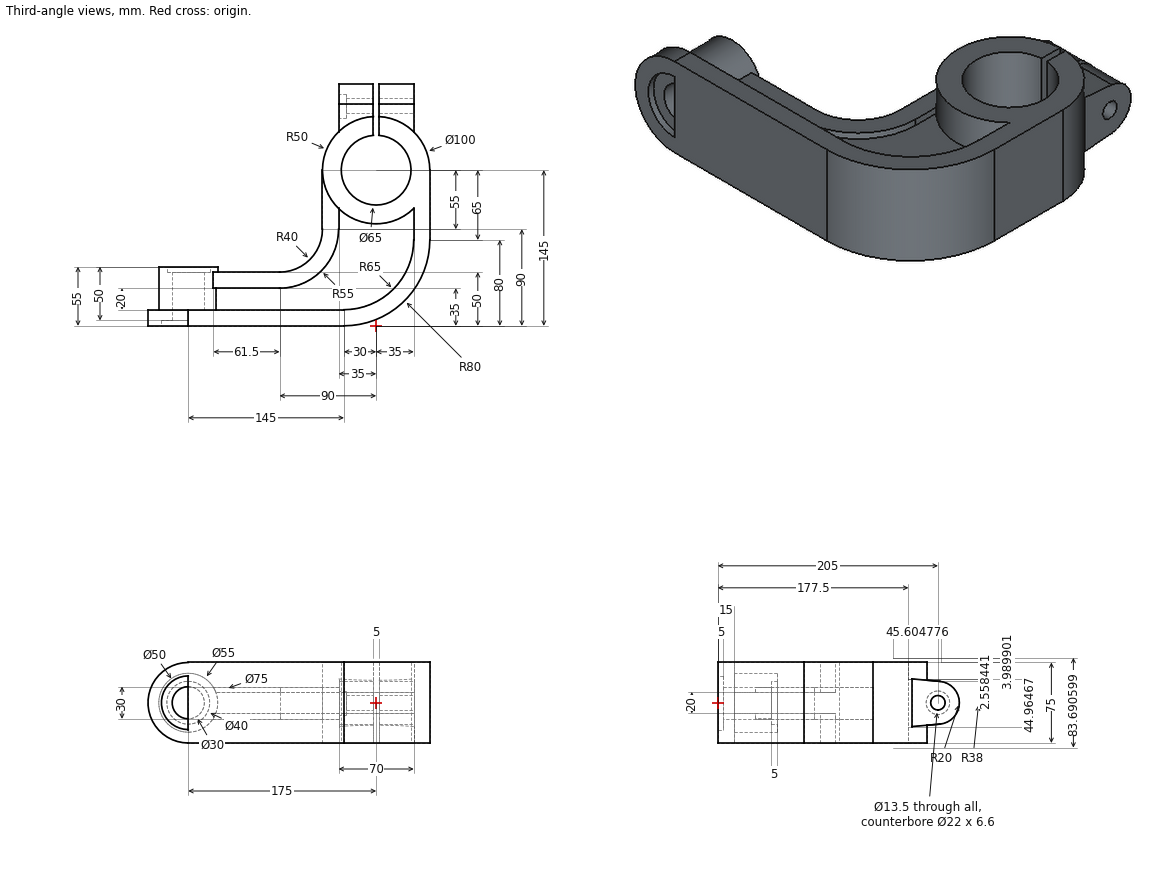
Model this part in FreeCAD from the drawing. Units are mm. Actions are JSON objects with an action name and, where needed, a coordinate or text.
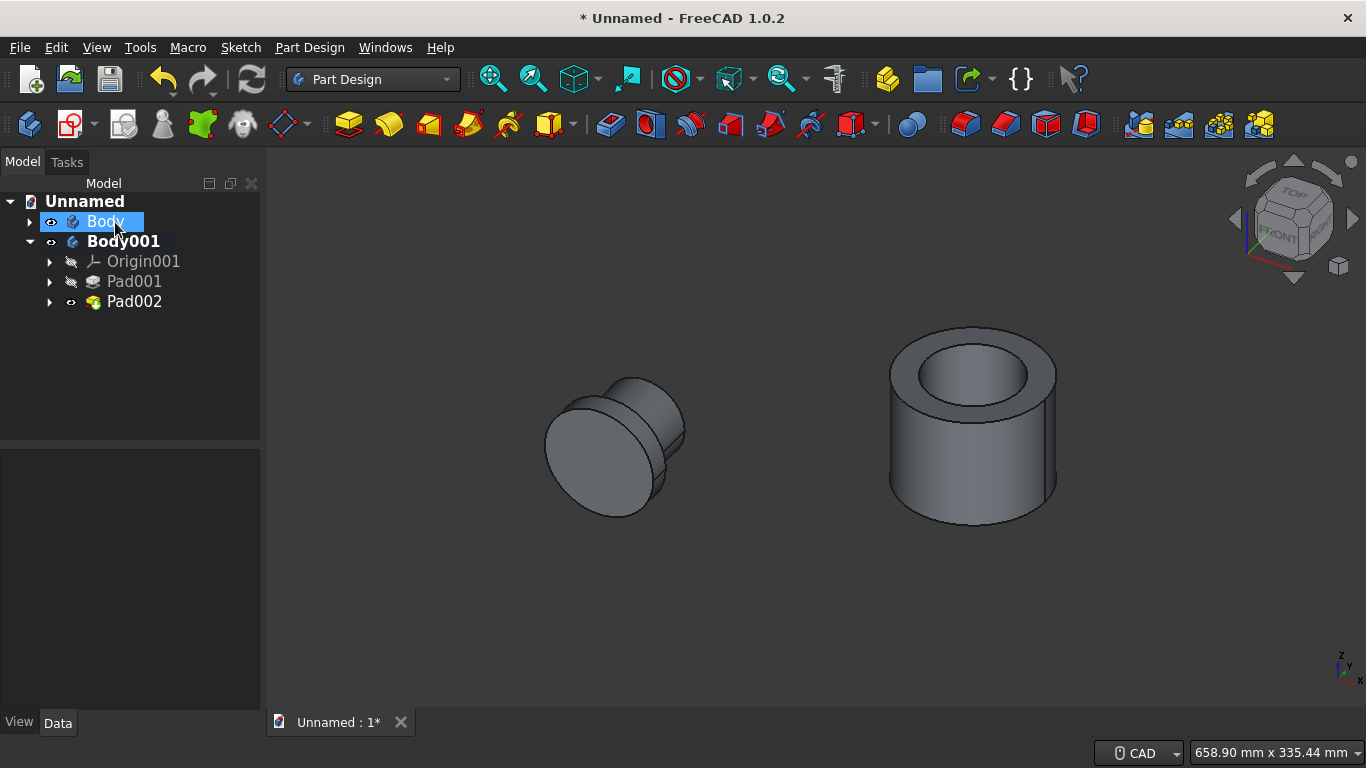
{"action": "left_click", "coordinate": [70, 124]}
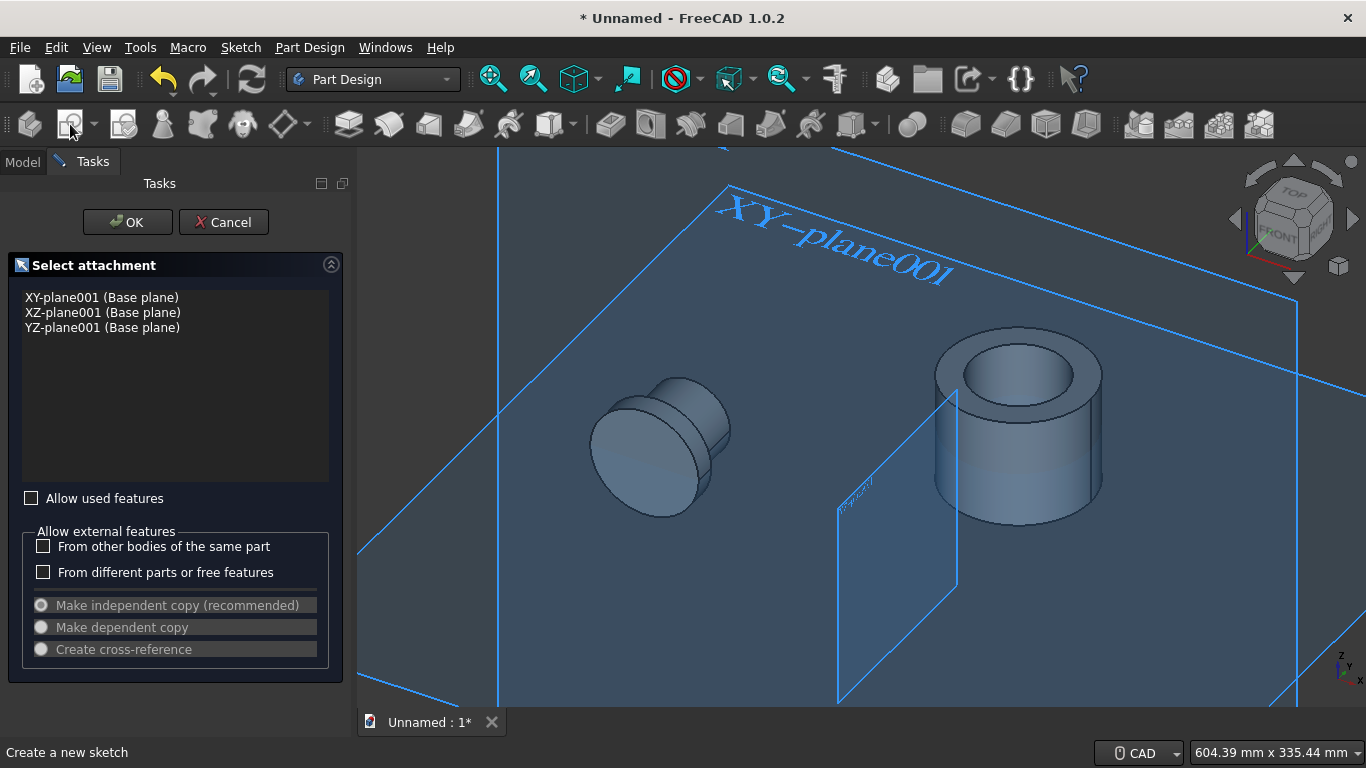
{"action": "left_click", "coordinate": [82, 312]}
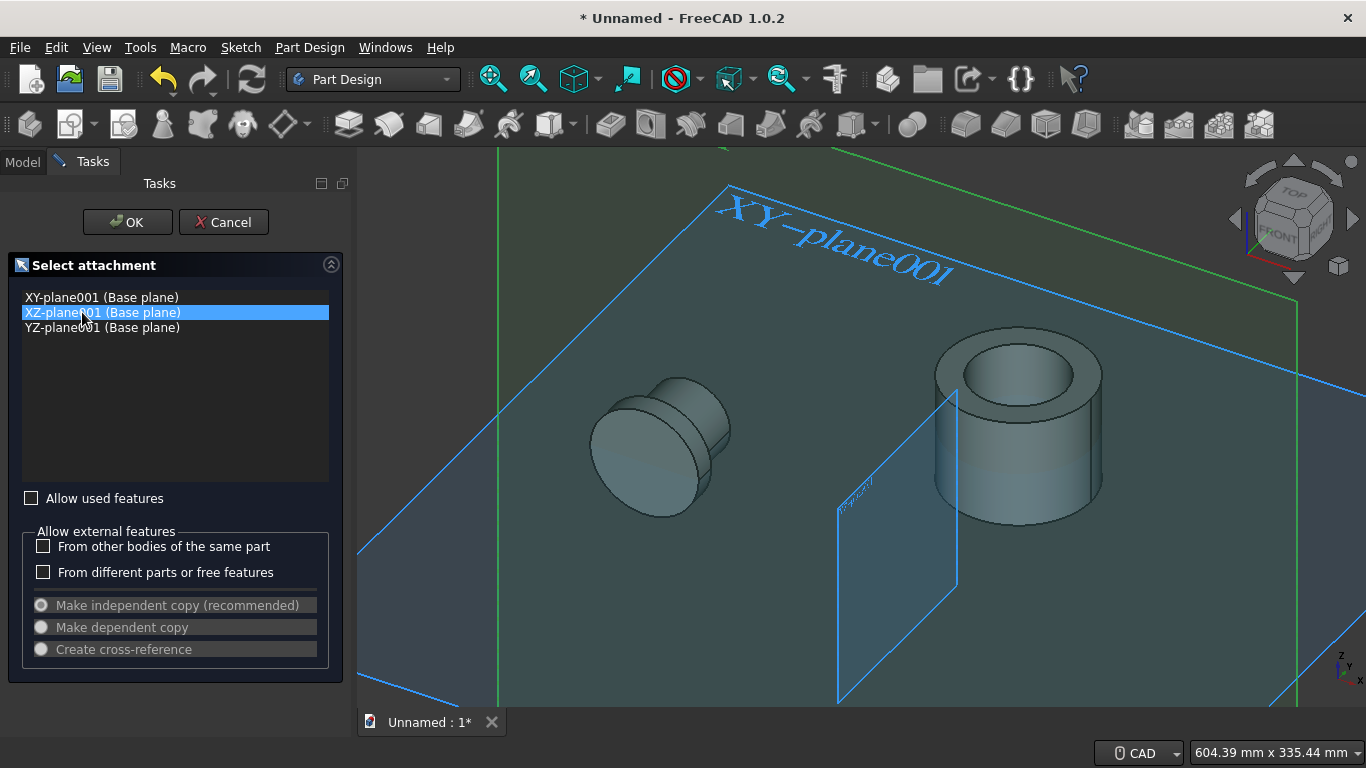
{"action": "left_click", "coordinate": [128, 222]}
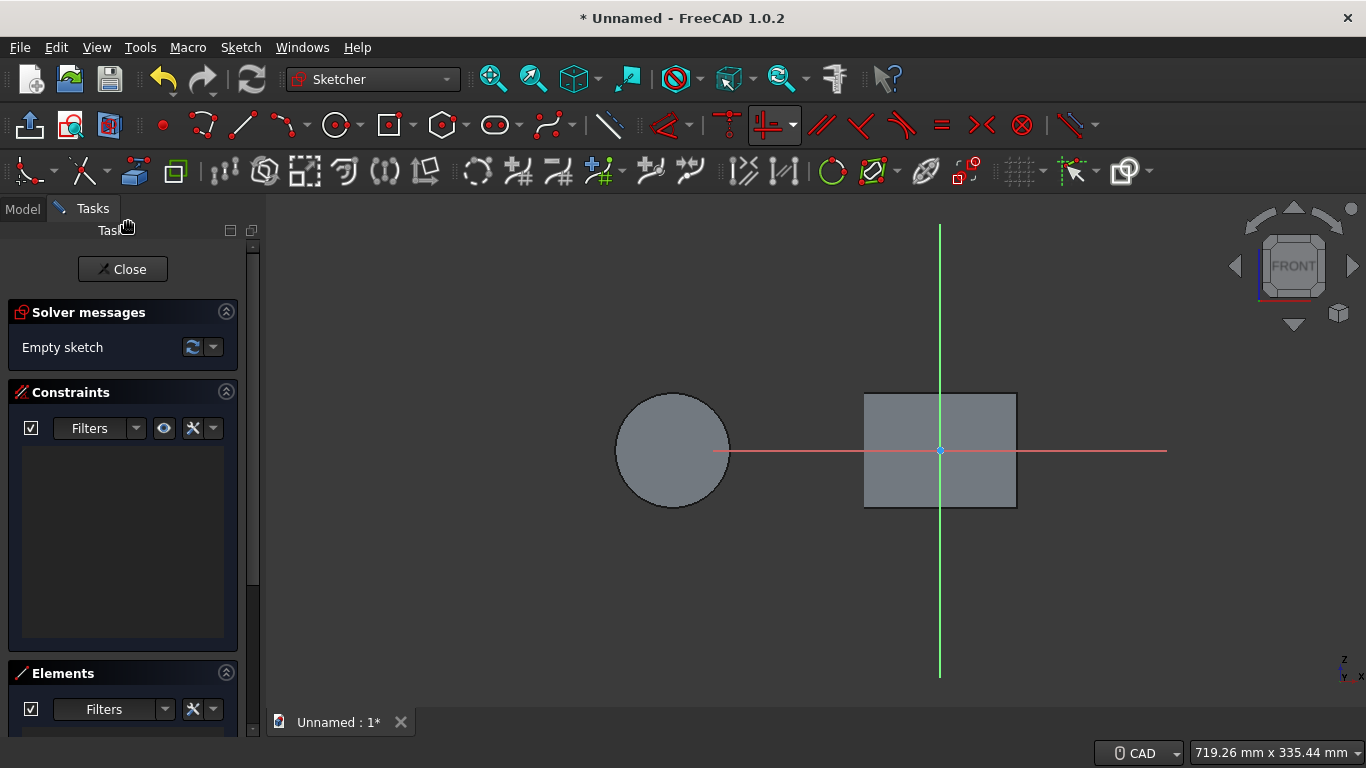
{"action": "scroll", "coordinate": [648, 450], "scroll_direction": "up", "scroll_amount": 7}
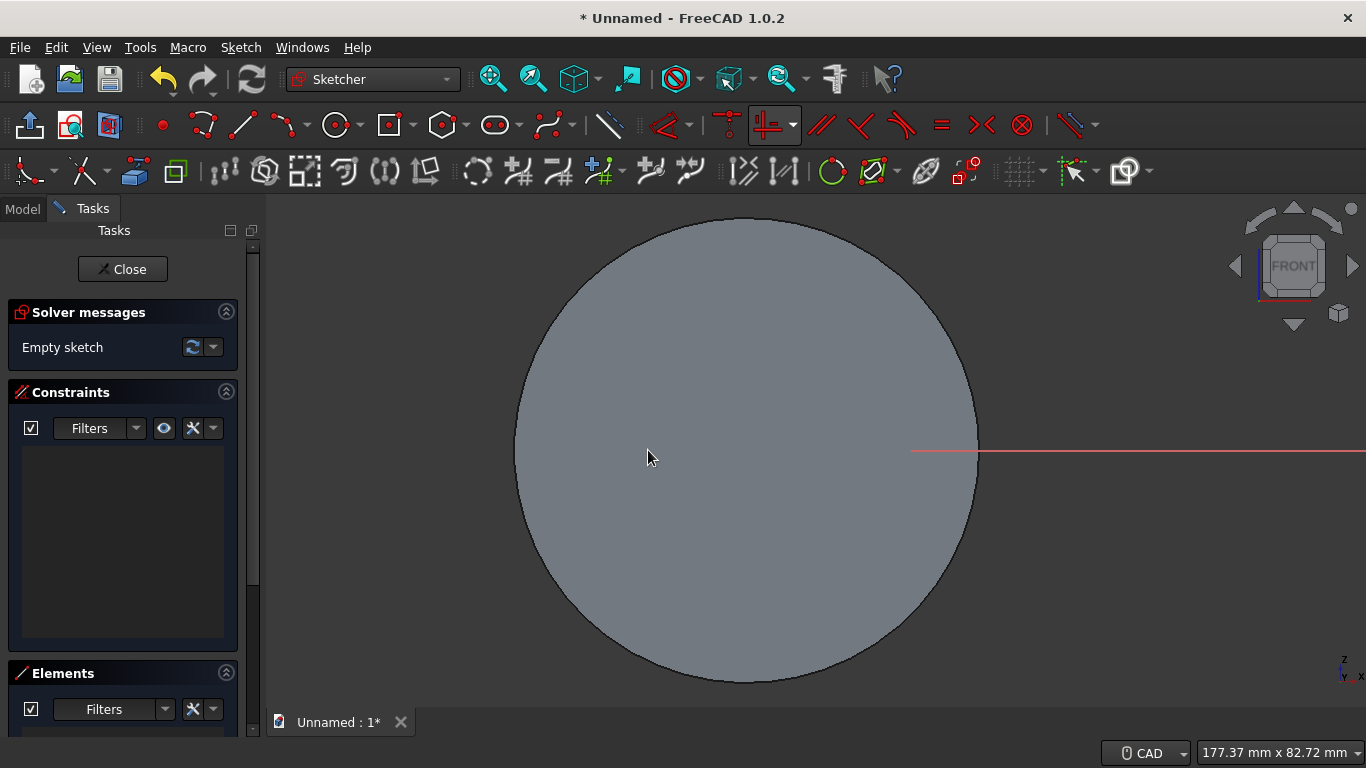
{"action": "key", "text": "g c"}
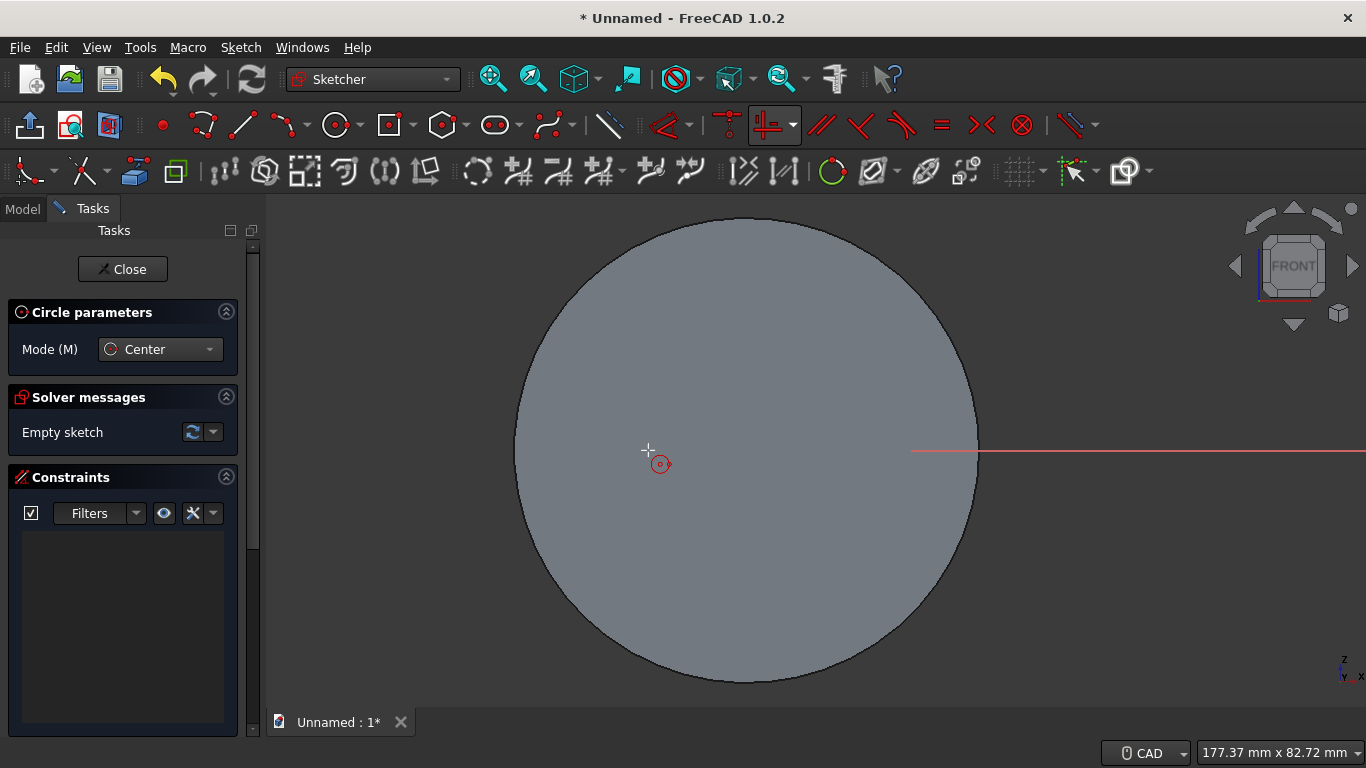
{"action": "left_click", "coordinate": [747, 450]}
{"action": "left_click", "coordinate": [856, 341]}
{"action": "key", "text": "Escape"}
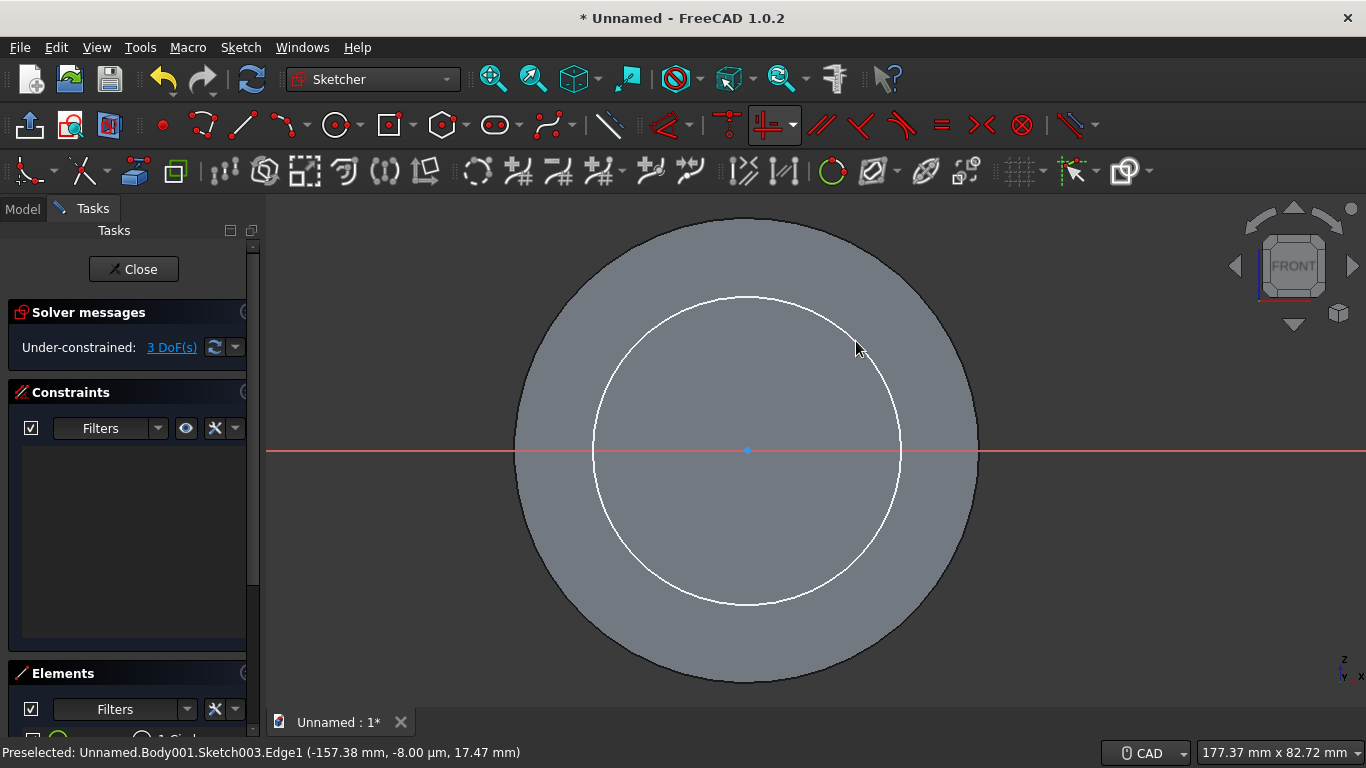
{"action": "left_click", "coordinate": [747, 451]}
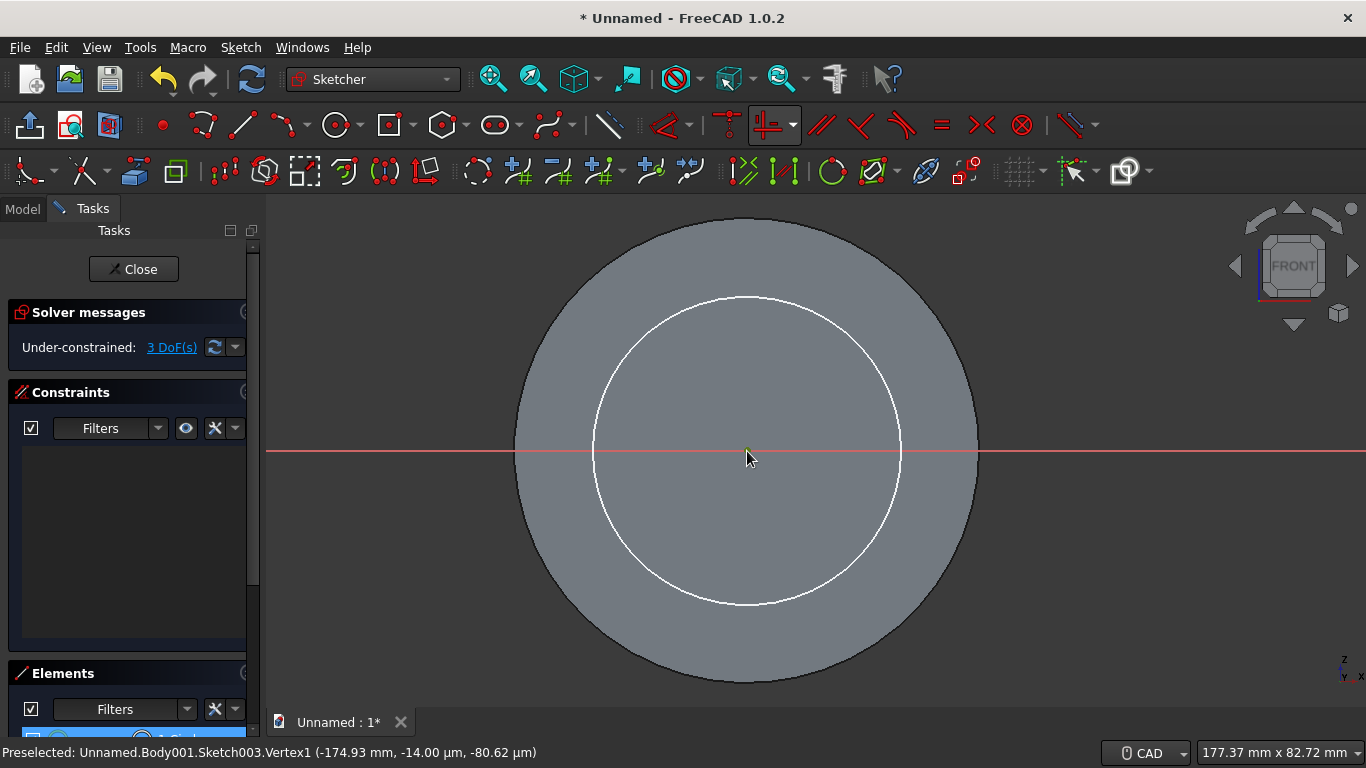
{"action": "left_click", "coordinate": [359, 450]}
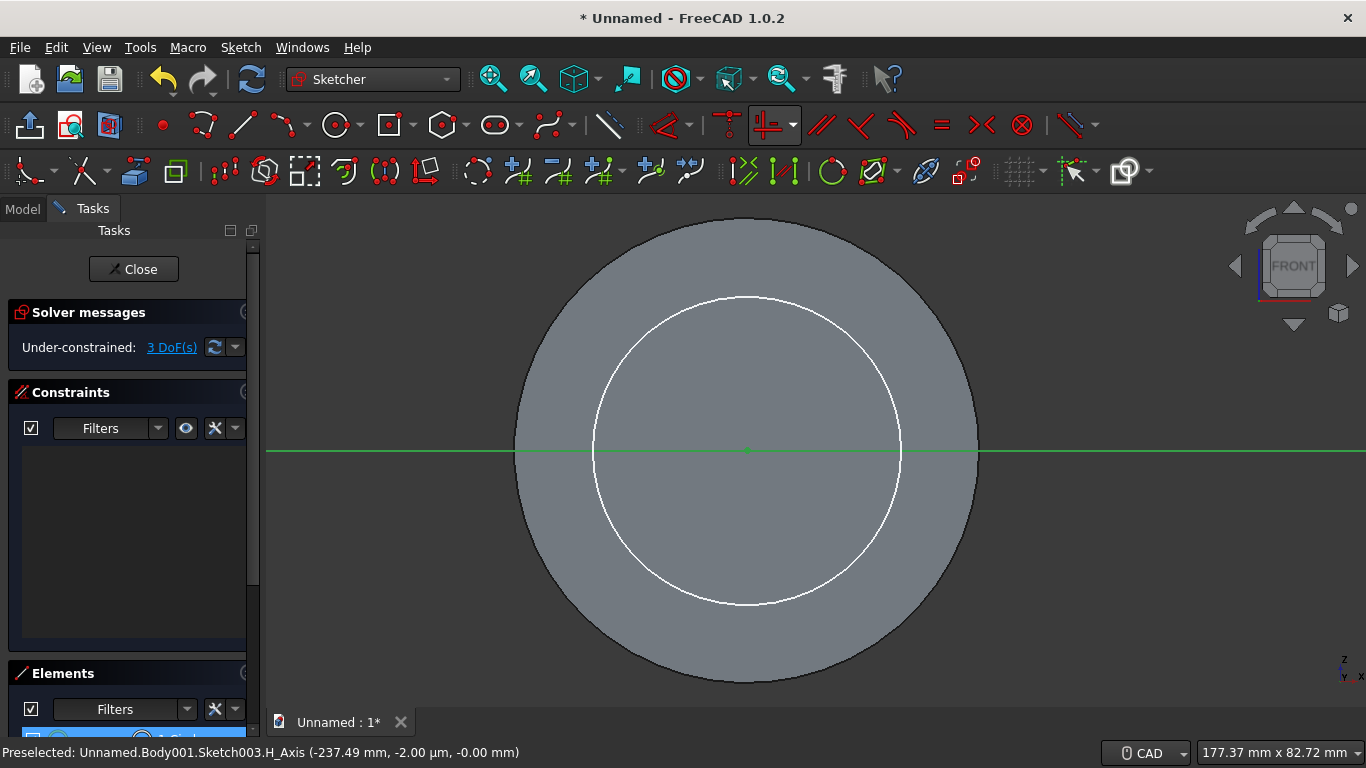
{"action": "key", "text": "c"}